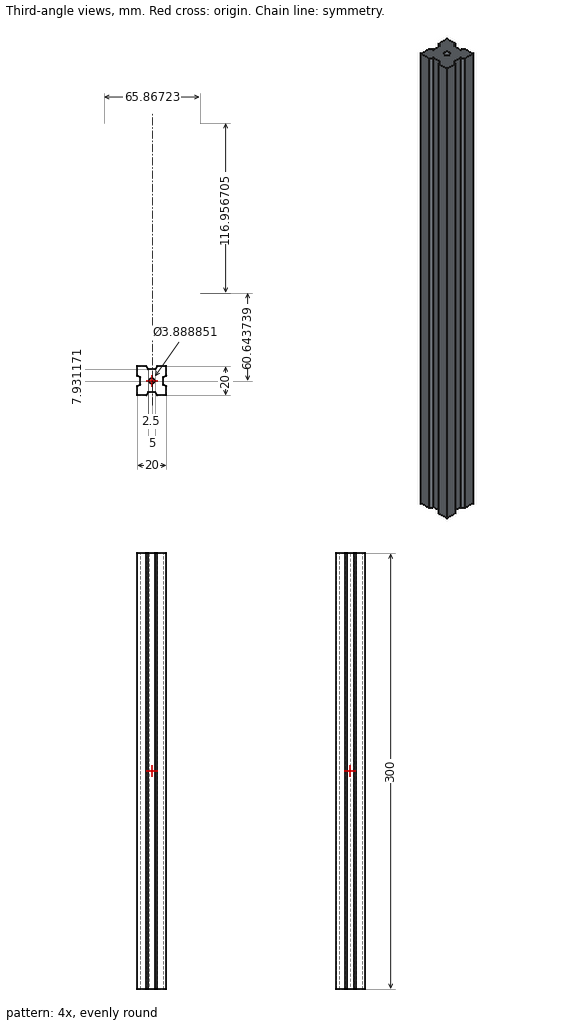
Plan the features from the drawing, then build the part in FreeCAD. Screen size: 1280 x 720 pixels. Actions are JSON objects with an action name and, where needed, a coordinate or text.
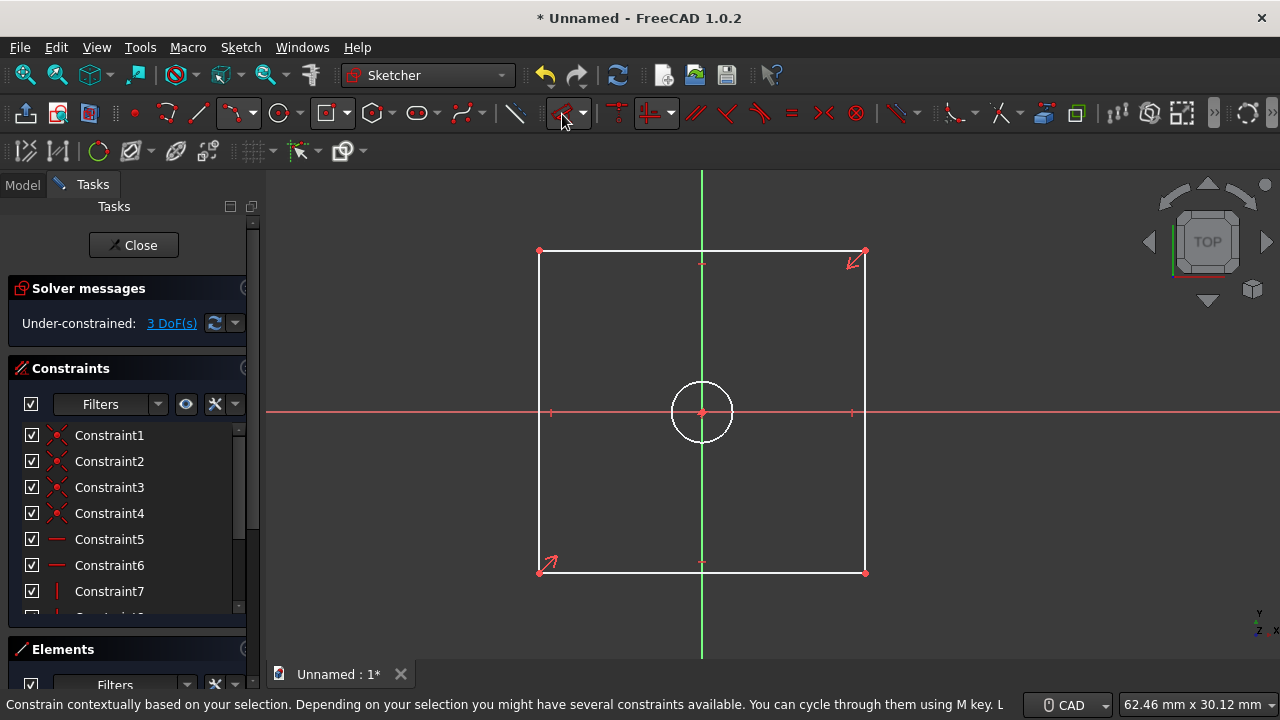
{"action": "left_click", "coordinate": [724, 391]}
{"action": "left_click", "coordinate": [747, 369]}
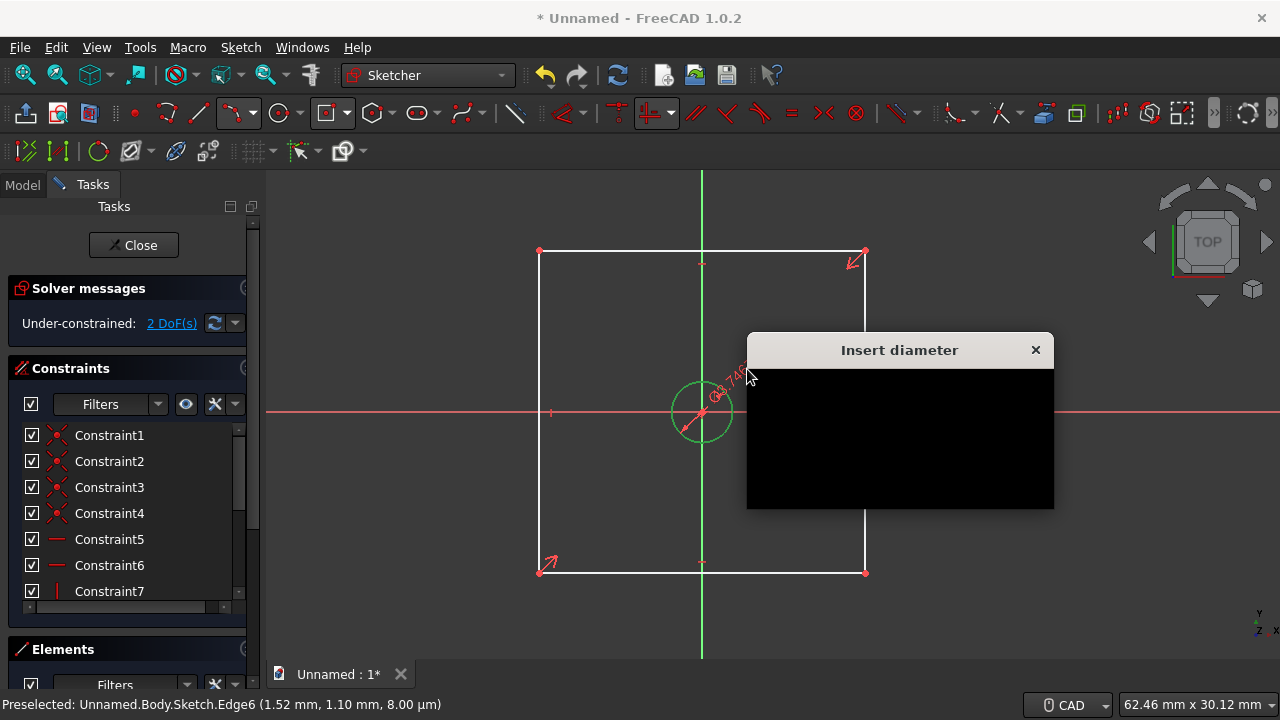
{"action": "type", "text": "3.888851"}
{"action": "key", "text": "Return"}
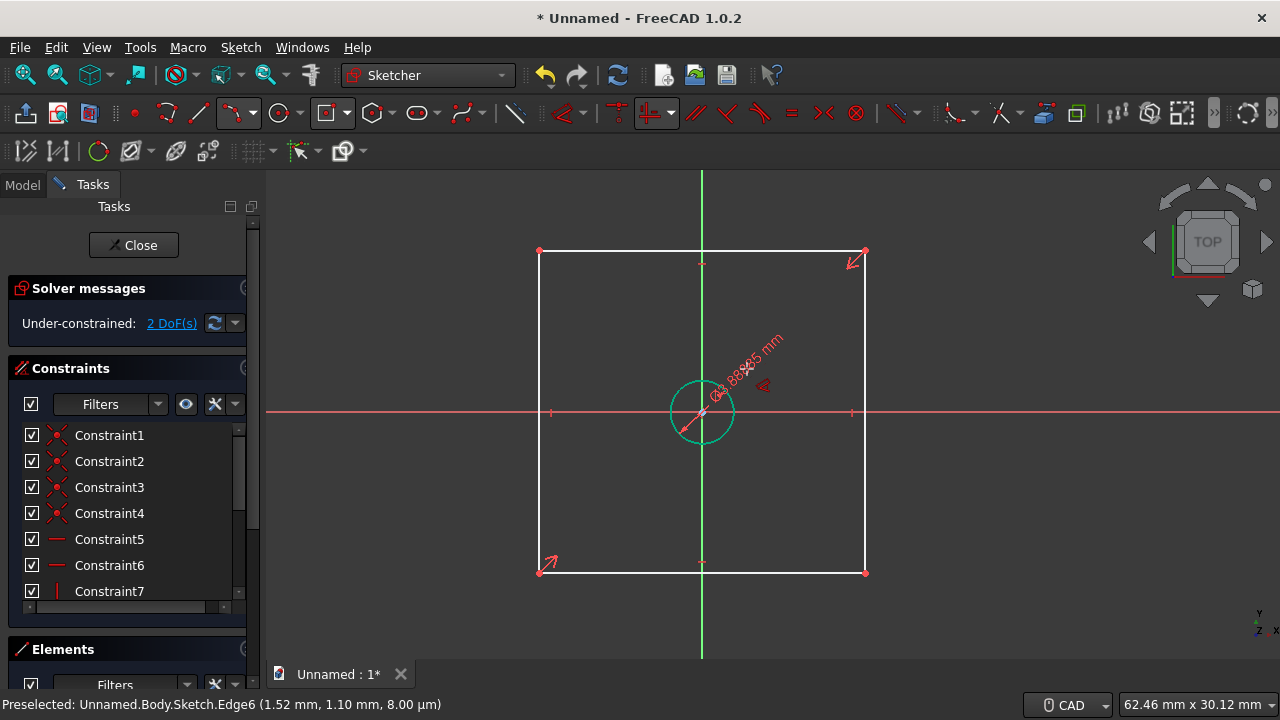
{"action": "left_click", "coordinate": [637, 573]}
{"action": "left_click", "coordinate": [627, 607]}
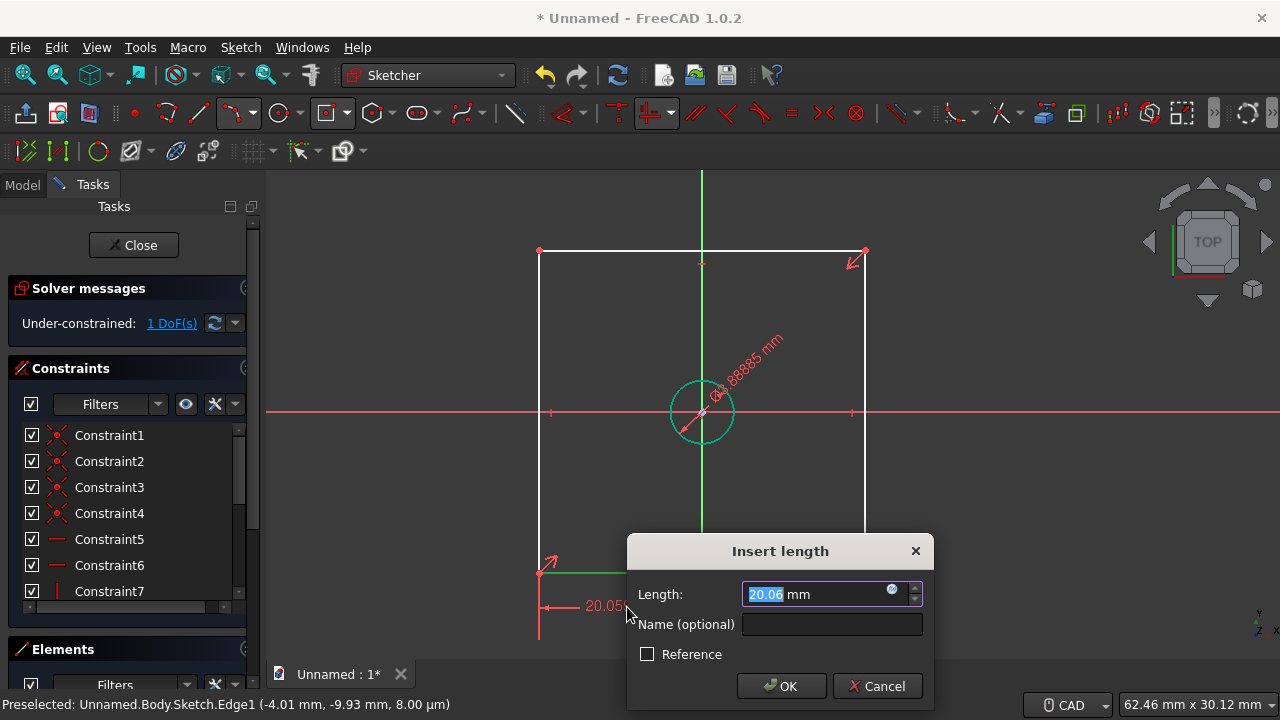
{"action": "type", "text": "20"}
{"action": "key", "text": "Return"}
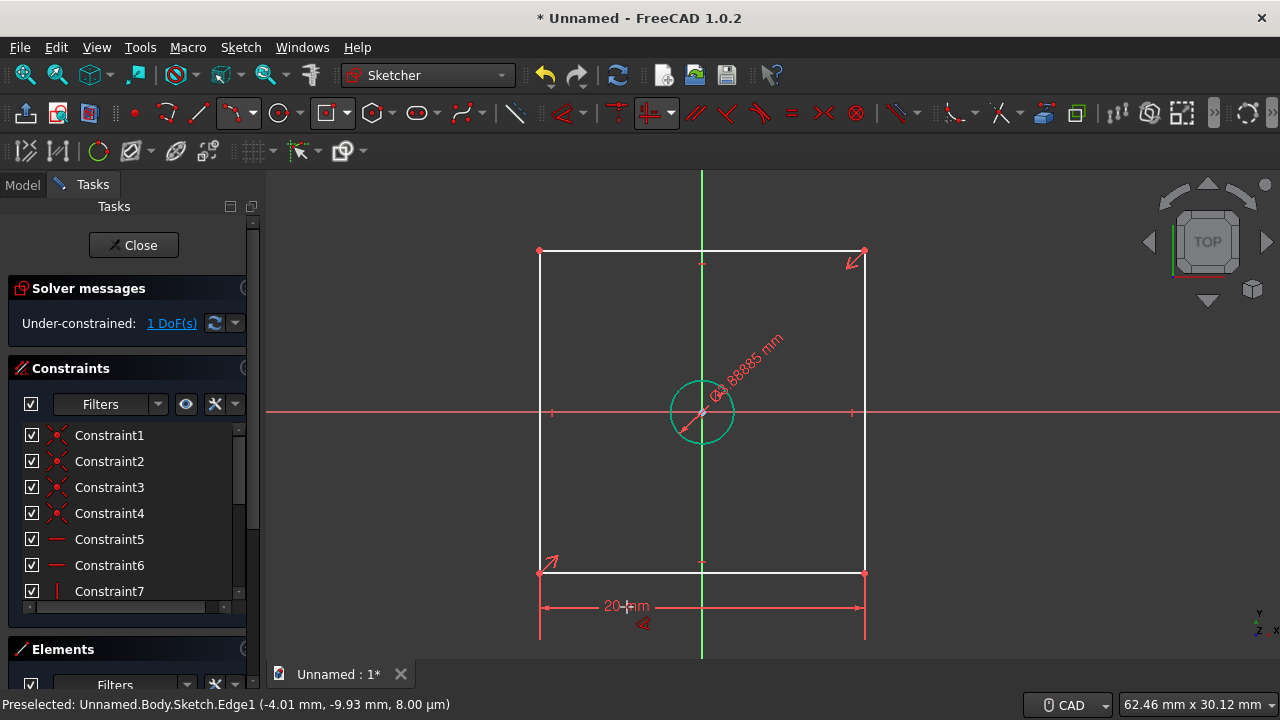
{"action": "left_click", "coordinate": [865, 477]}
{"action": "left_click", "coordinate": [899, 338]}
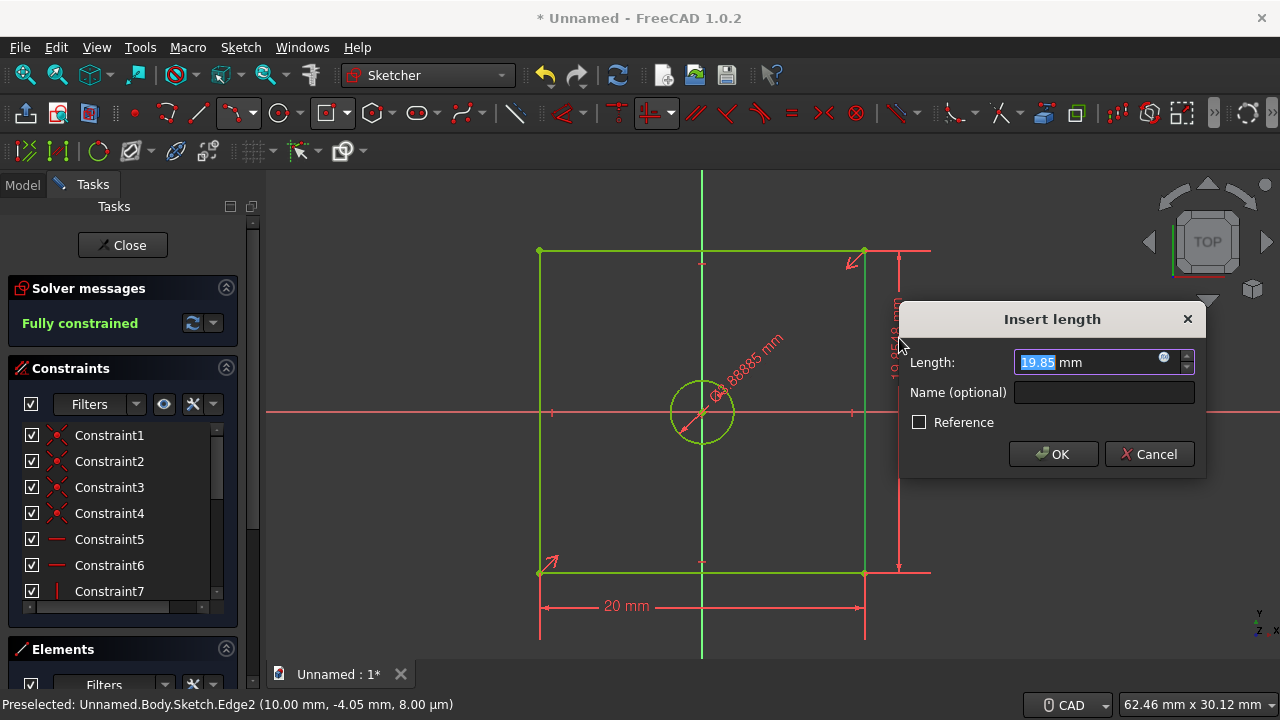
{"action": "type", "text": "20"}
{"action": "key", "text": "Return"}
{"action": "key", "text": "Escape"}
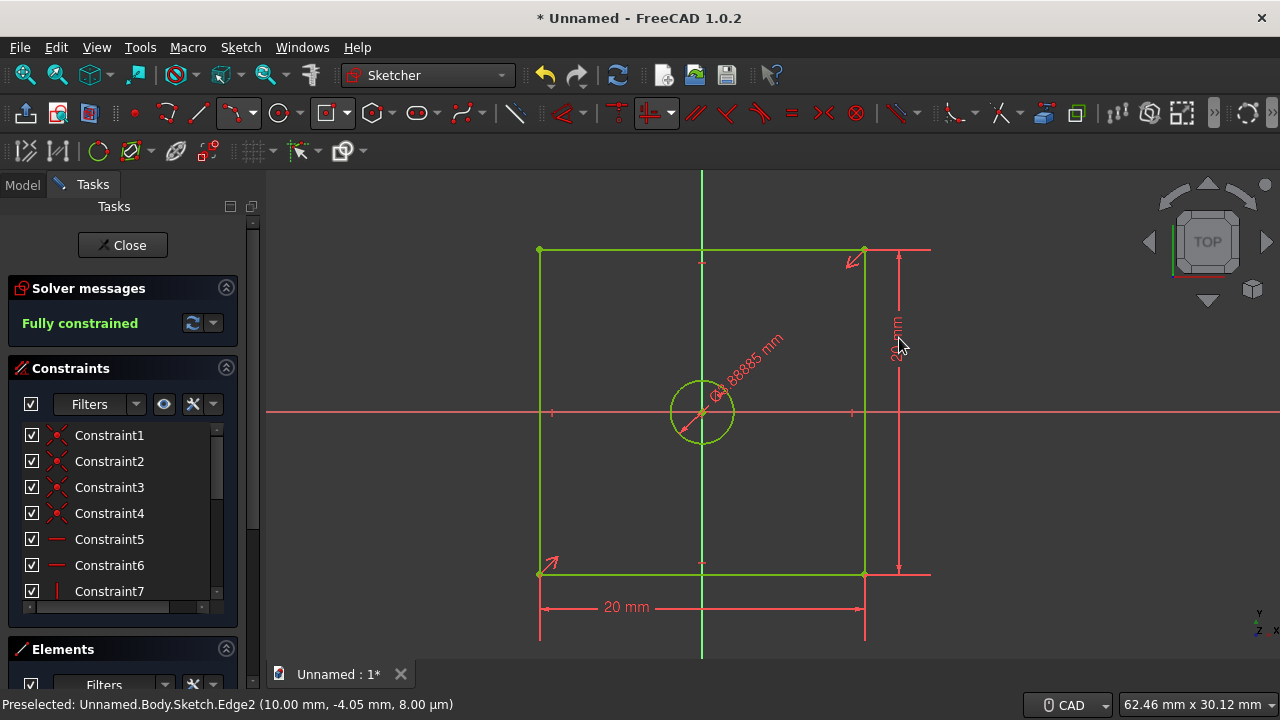
{"action": "left_click", "coordinate": [123, 245]}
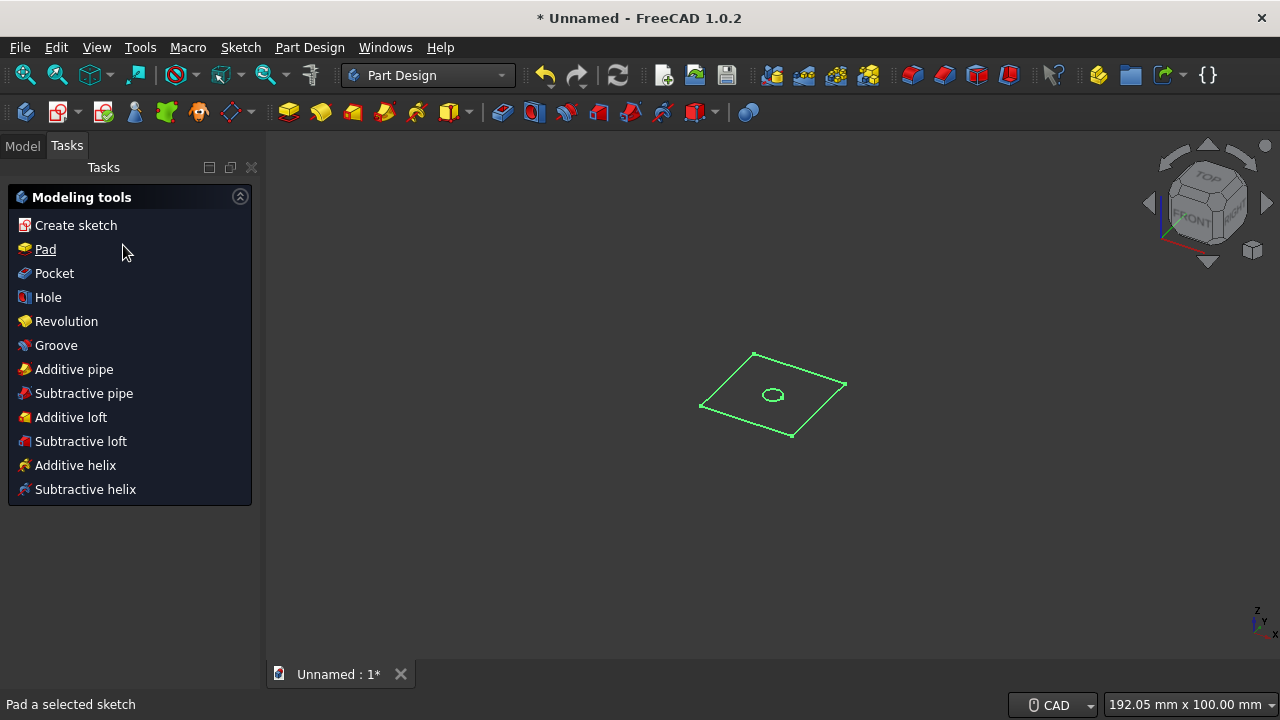
{"action": "left_click", "coordinate": [290, 112]}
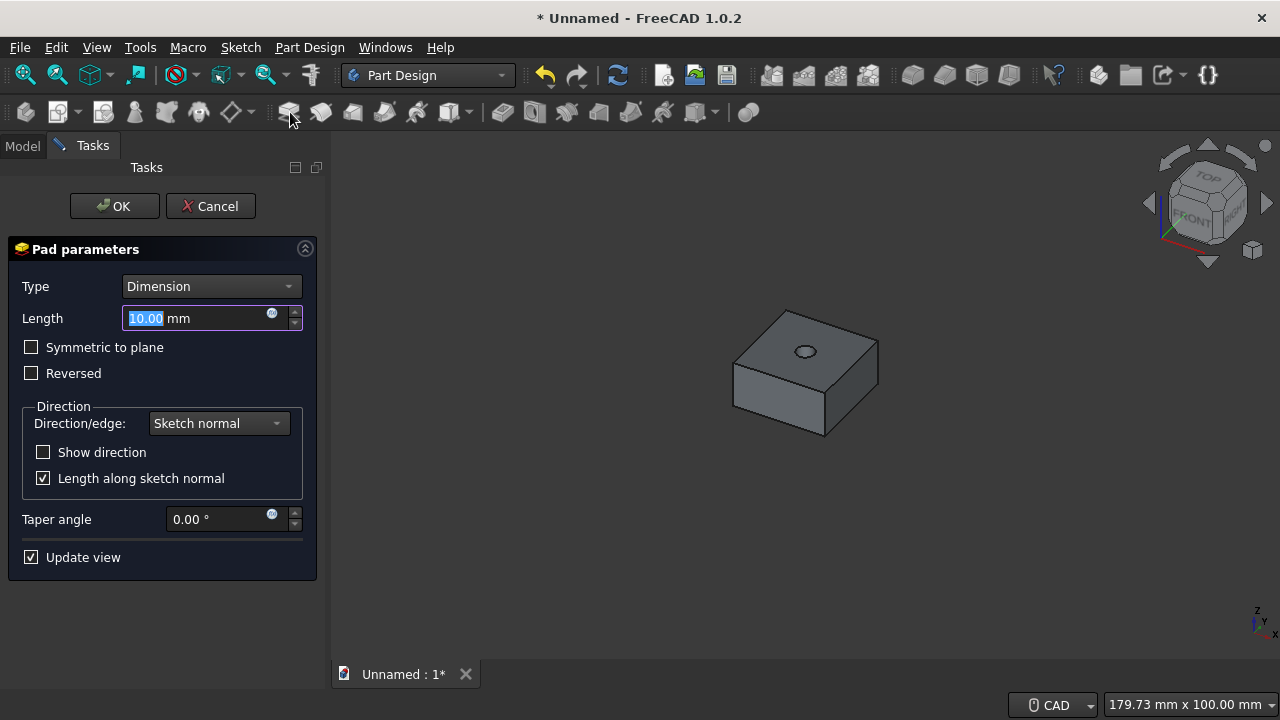
{"action": "type", "text": "300"}
{"action": "key", "text": "Tab"}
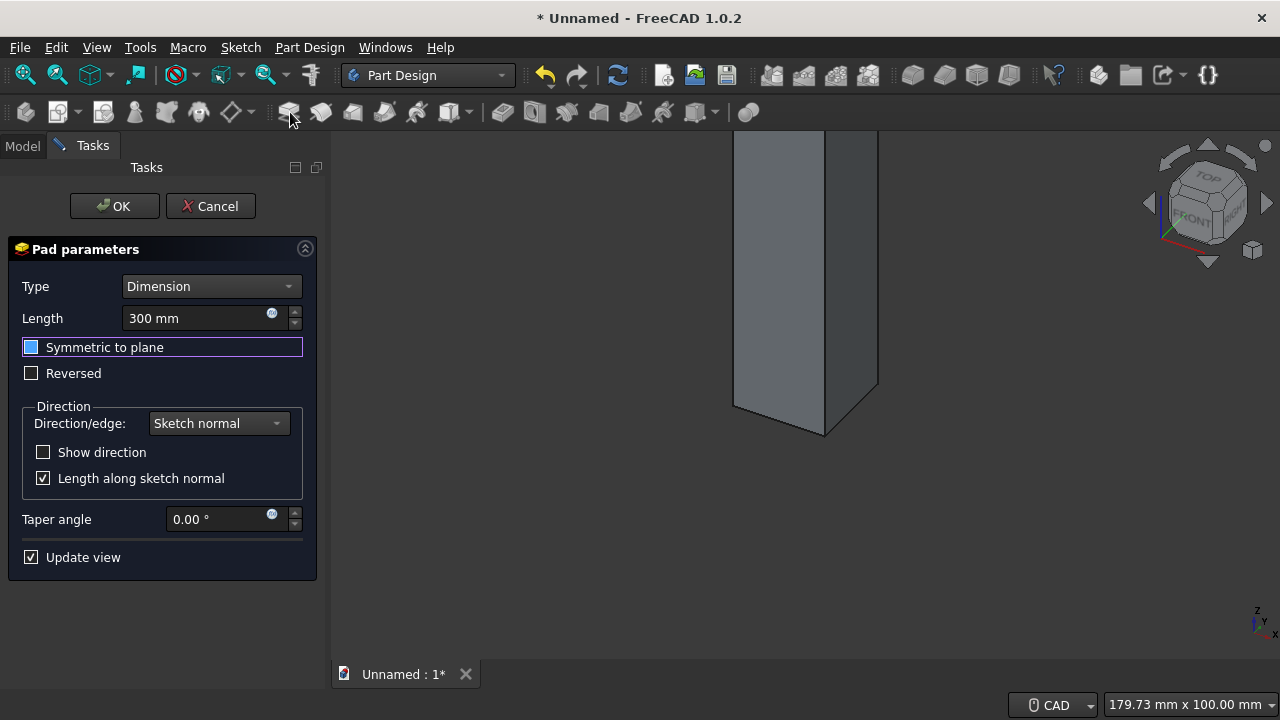
{"action": "left_click", "coordinate": [30, 347]}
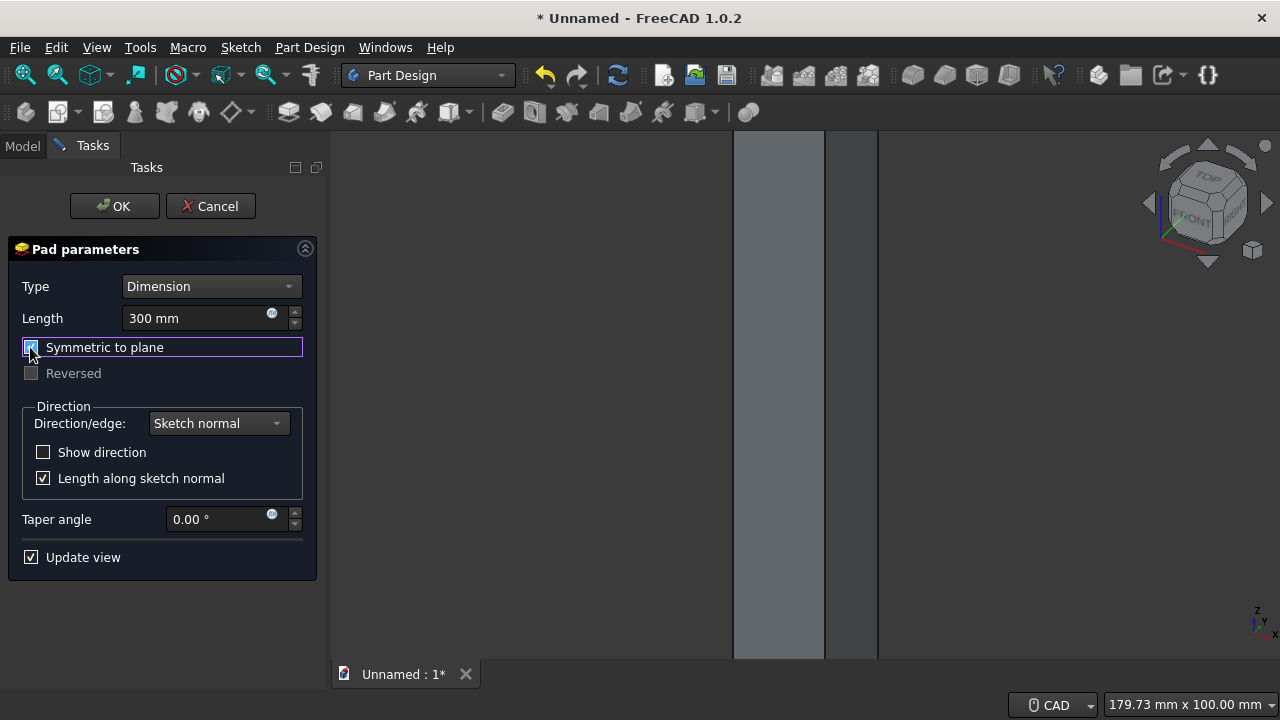
{"action": "left_click", "coordinate": [115, 206]}